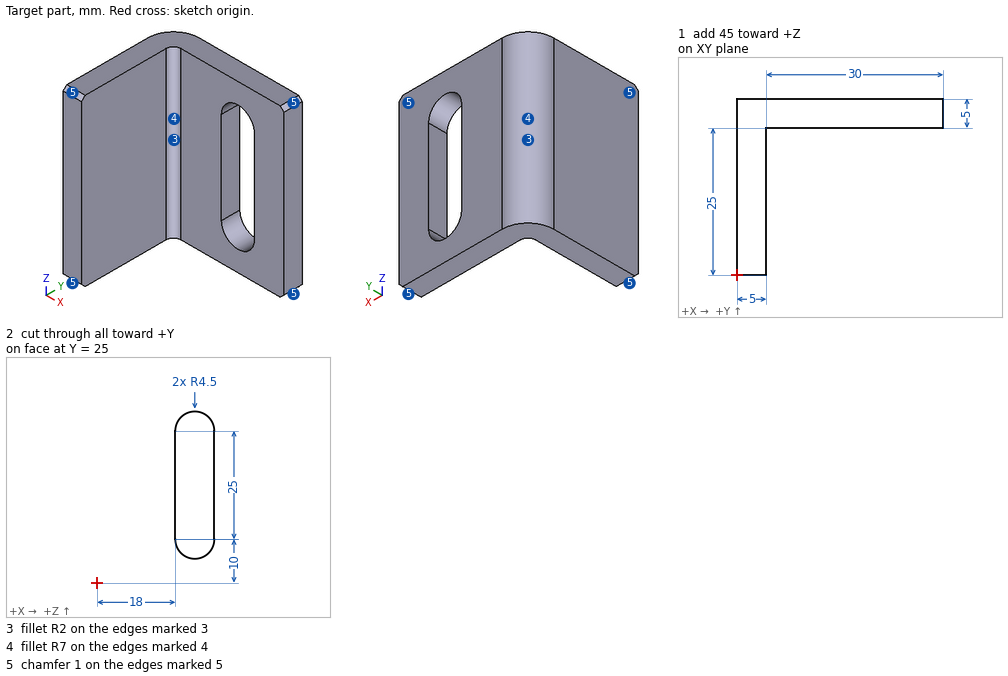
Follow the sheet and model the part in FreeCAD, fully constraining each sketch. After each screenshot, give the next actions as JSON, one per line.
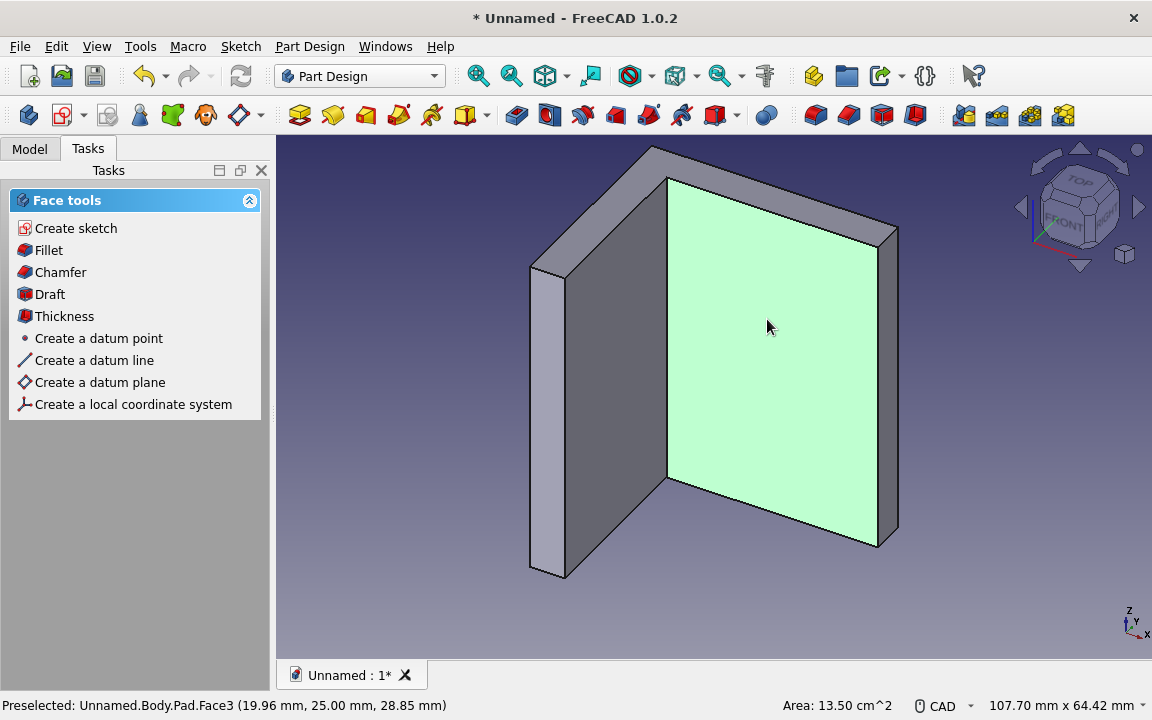
{"action": "left_click", "coordinate": [62, 116]}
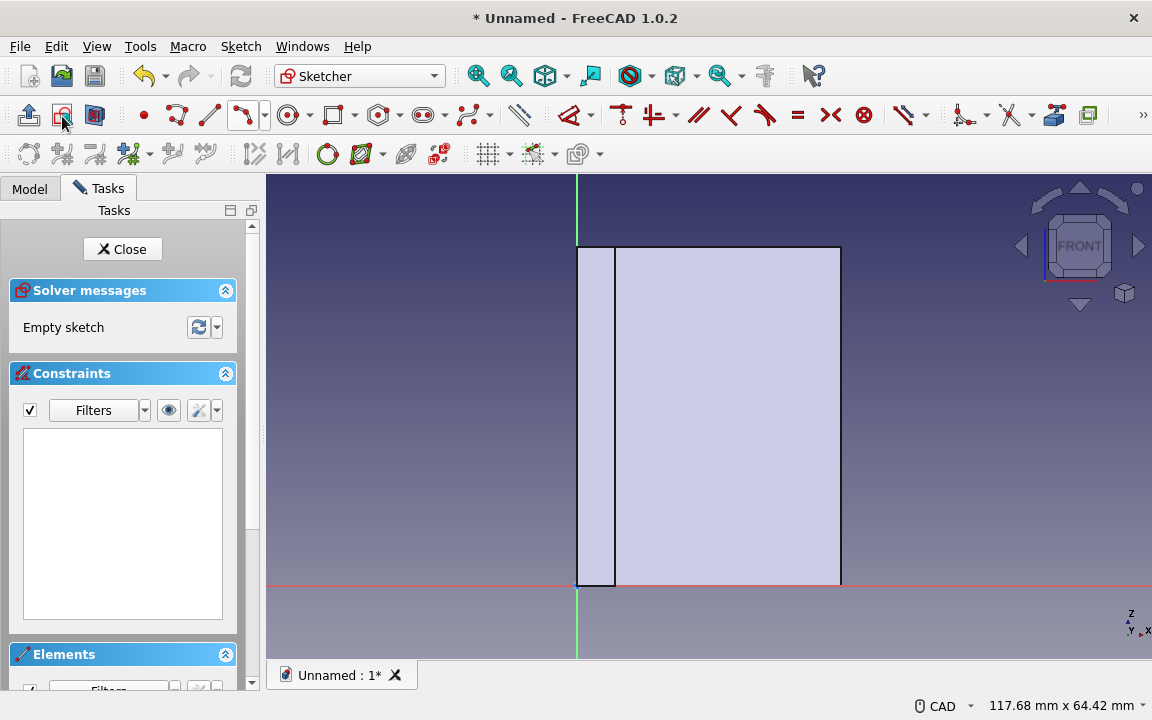
{"action": "key", "text": "q s"}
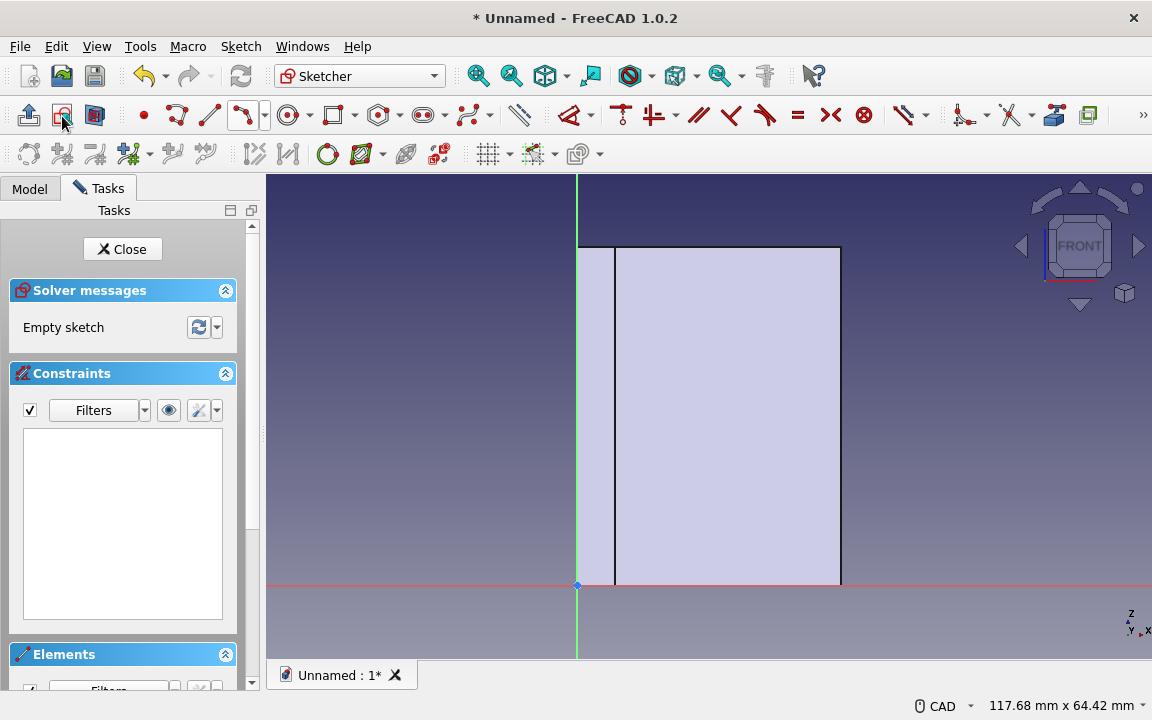
{"action": "key", "text": "g s"}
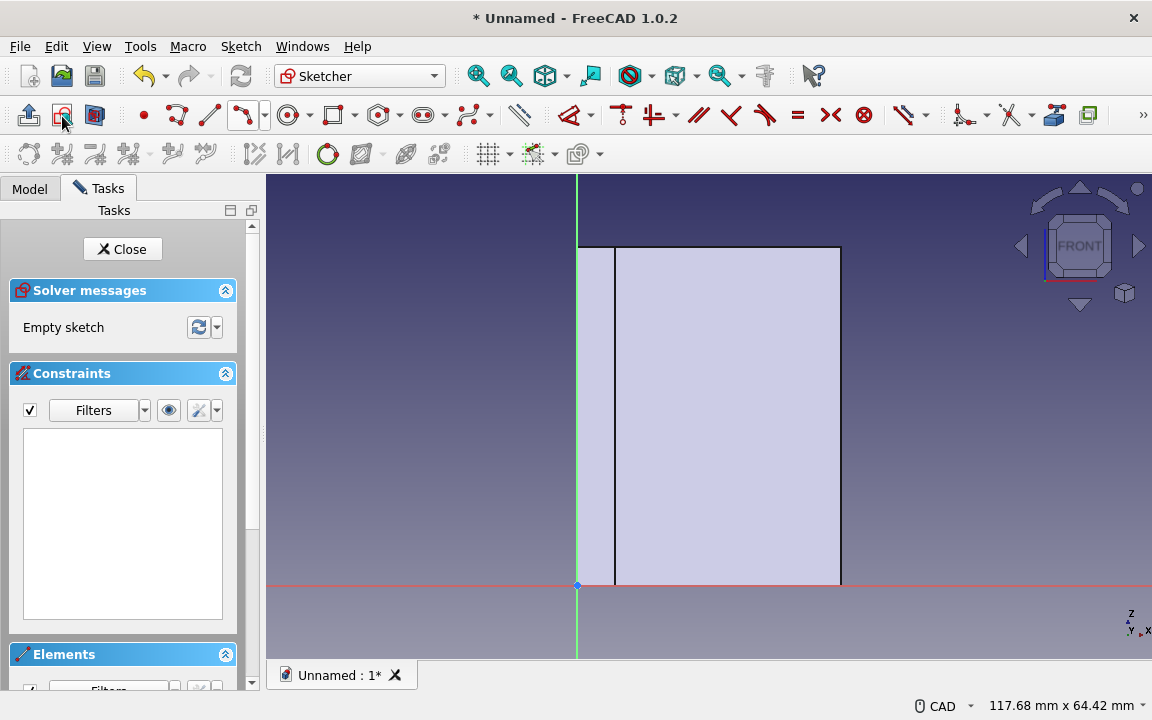
{"action": "left_click", "coordinate": [747, 511]}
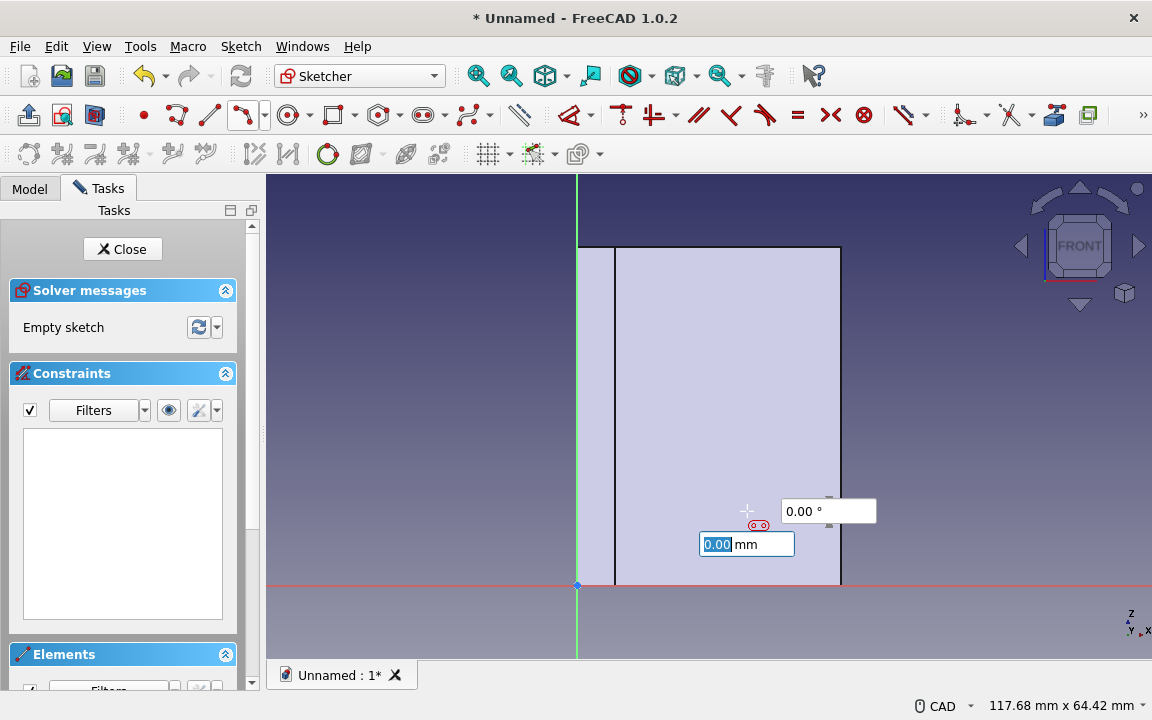
{"action": "left_click", "coordinate": [747, 322]}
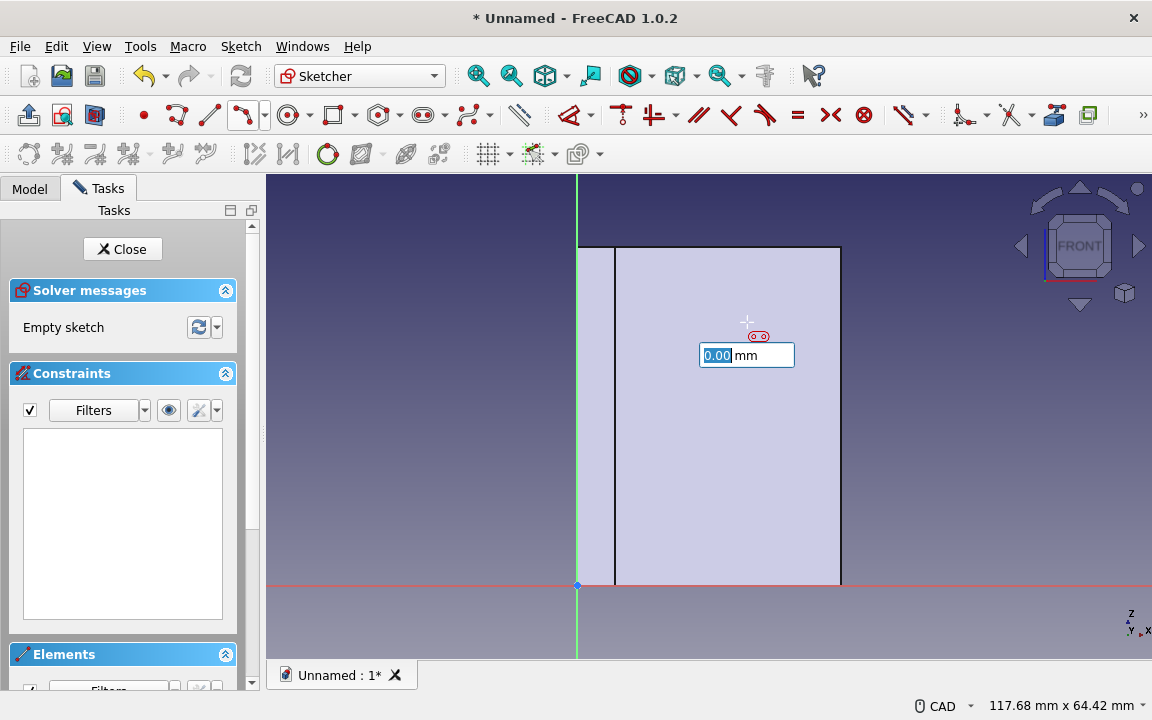
{"action": "left_click", "coordinate": [781, 417]}
{"action": "key", "text": "Escape"}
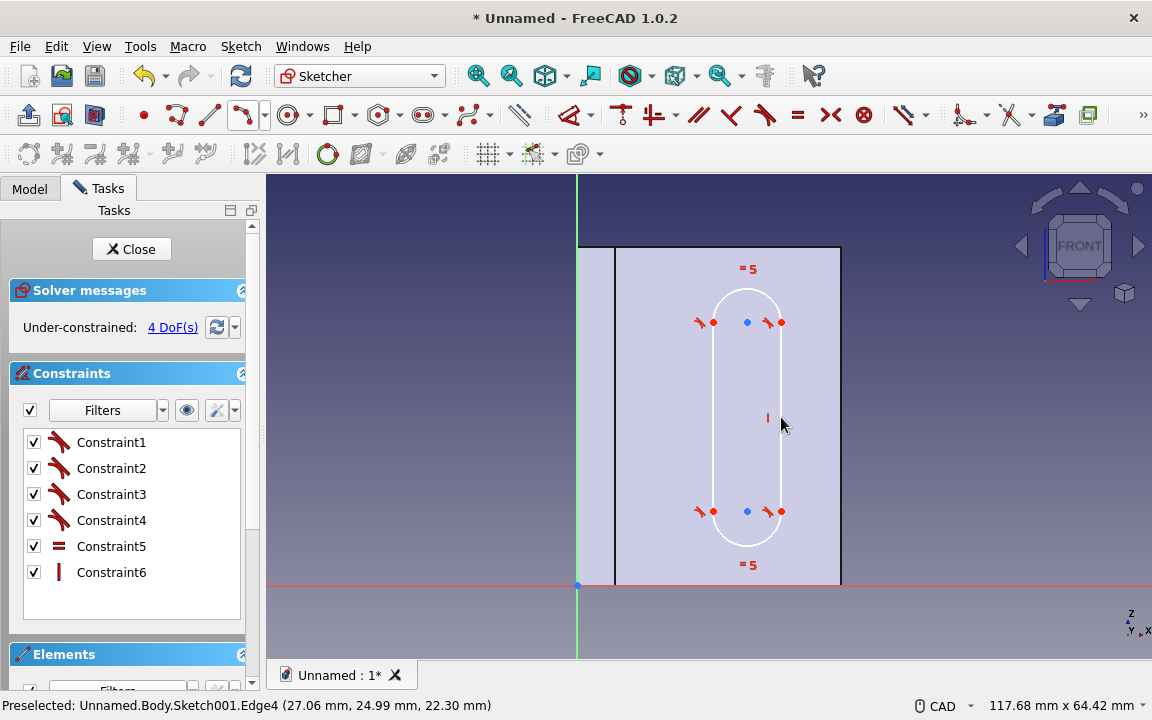
{"action": "left_click", "coordinate": [568, 116]}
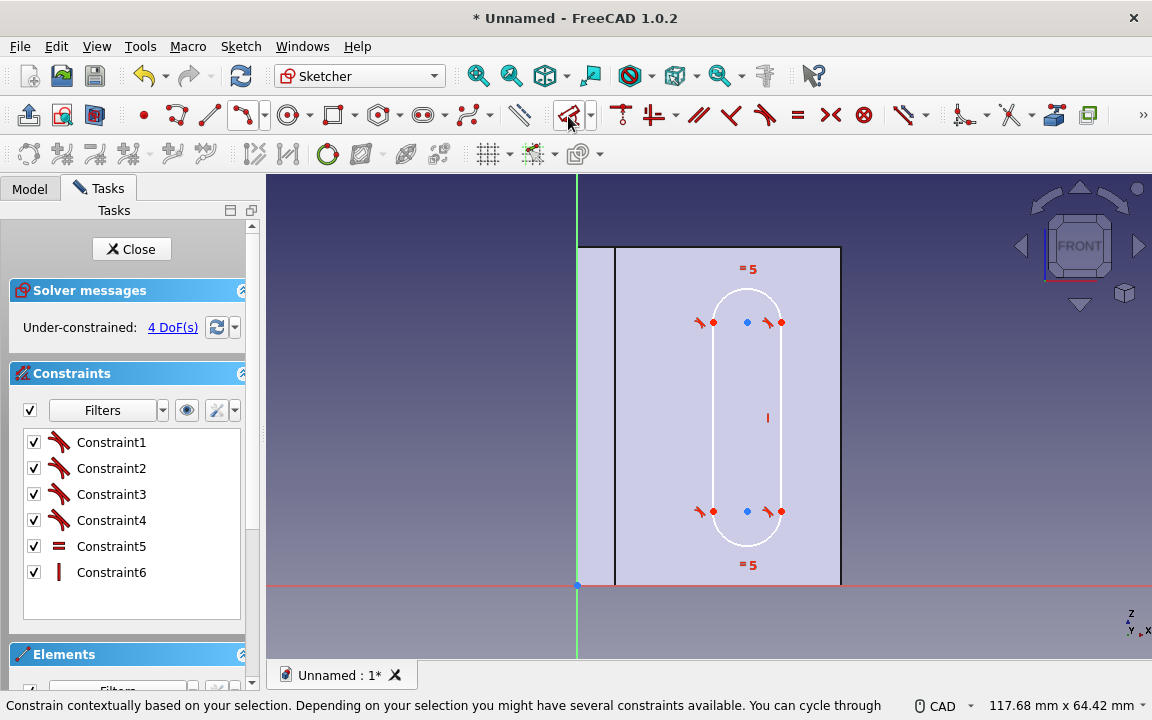
{"action": "left_click", "coordinate": [727, 540]}
{"action": "left_click", "coordinate": [708, 566]}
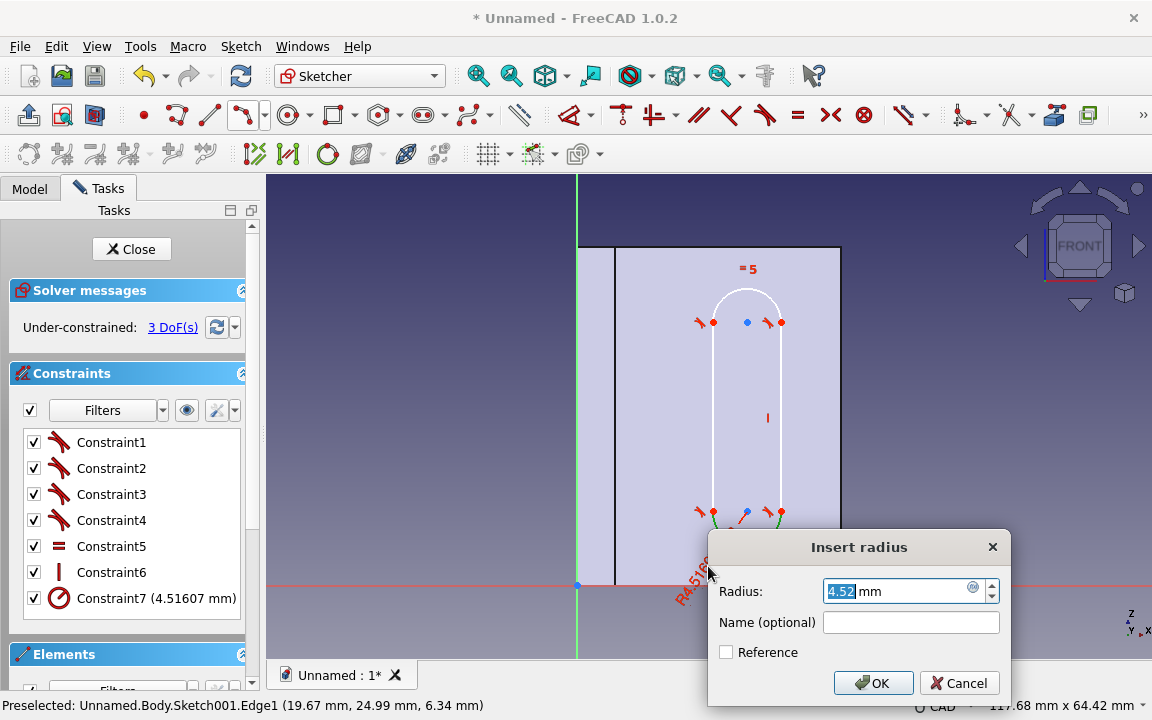
{"action": "type", "text": "4.5"}
{"action": "key", "text": "Return"}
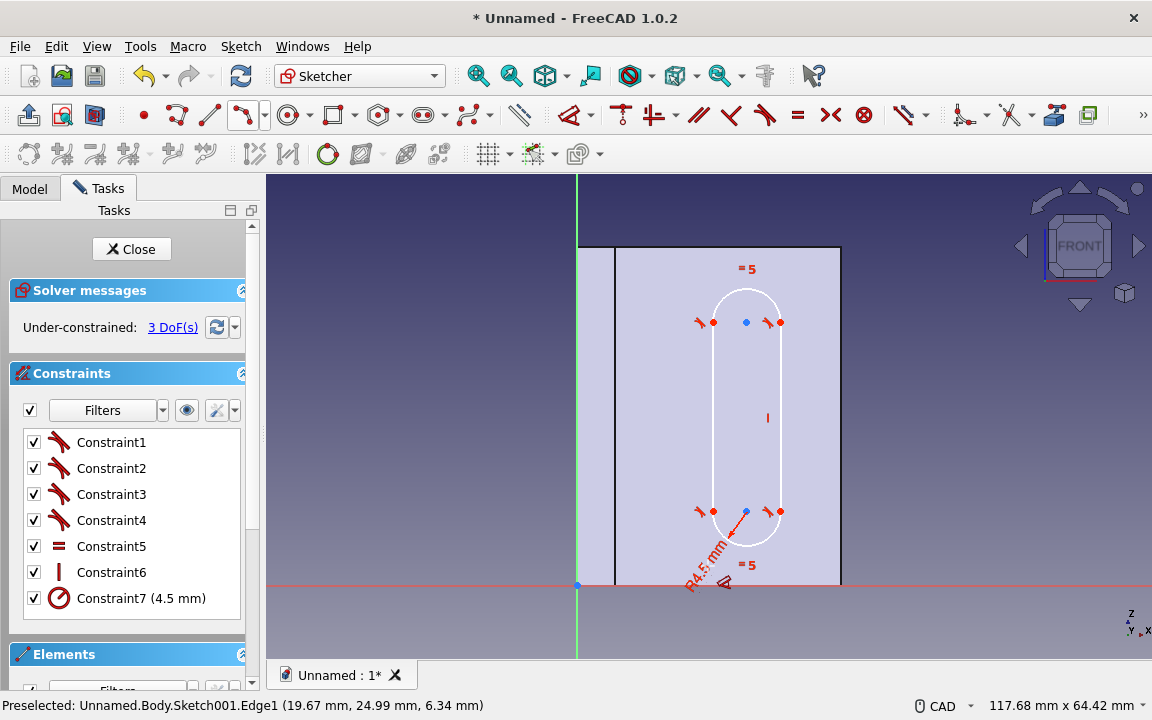
{"action": "left_click", "coordinate": [713, 455]}
{"action": "left_click", "coordinate": [747, 417]}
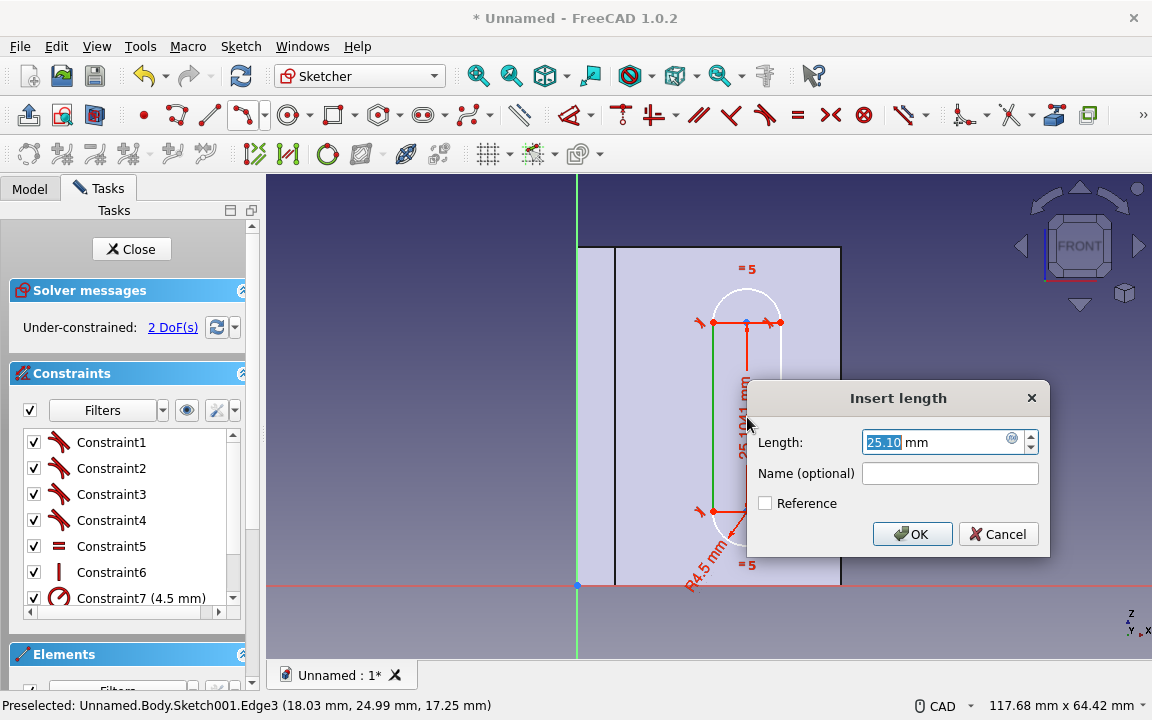
{"action": "type", "text": "25"}
{"action": "key", "text": "Return"}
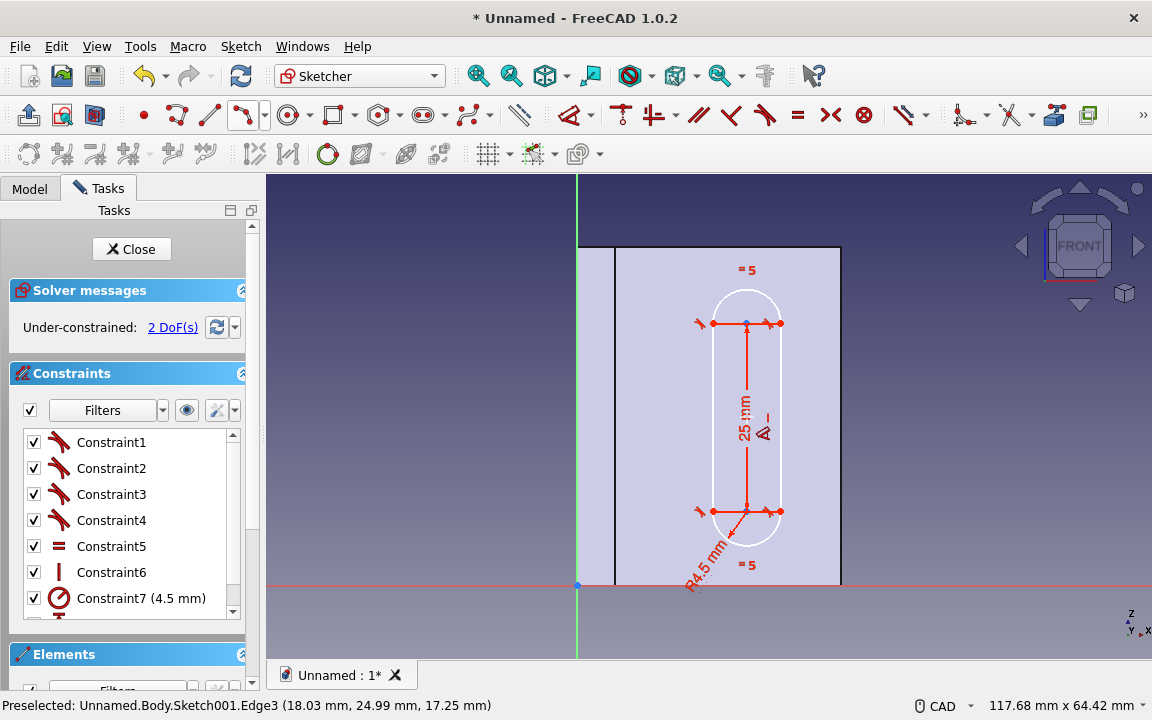
{"action": "left_click", "coordinate": [713, 512]}
{"action": "left_click", "coordinate": [645, 620]}